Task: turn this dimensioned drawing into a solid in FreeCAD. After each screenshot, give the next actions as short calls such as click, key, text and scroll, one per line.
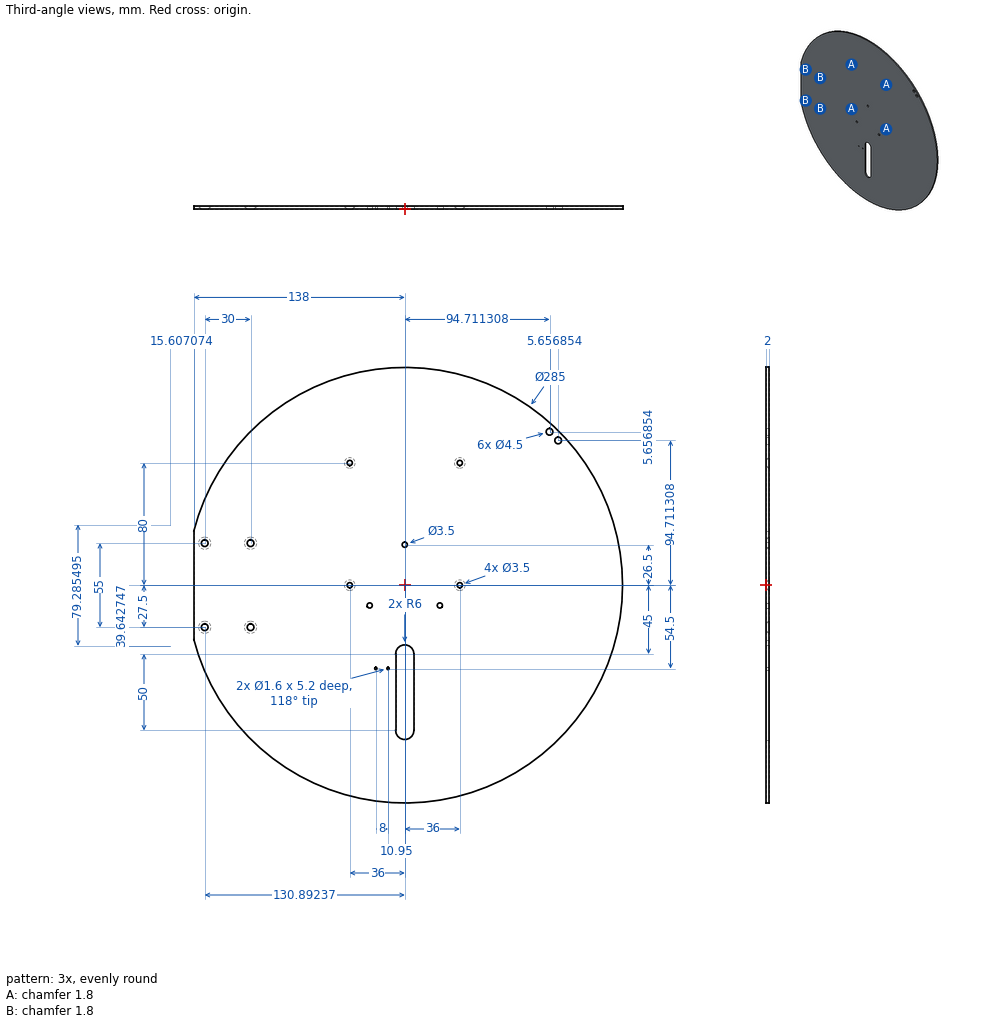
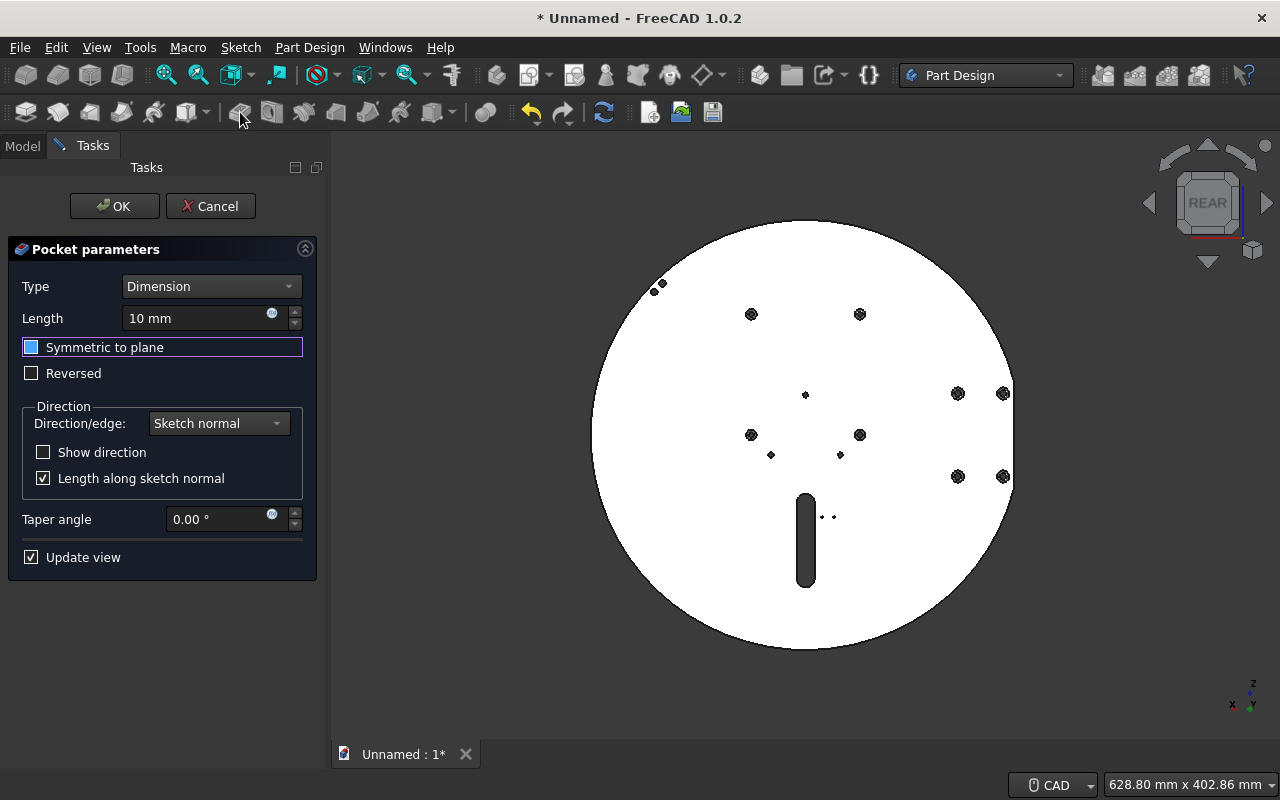
click(115, 206)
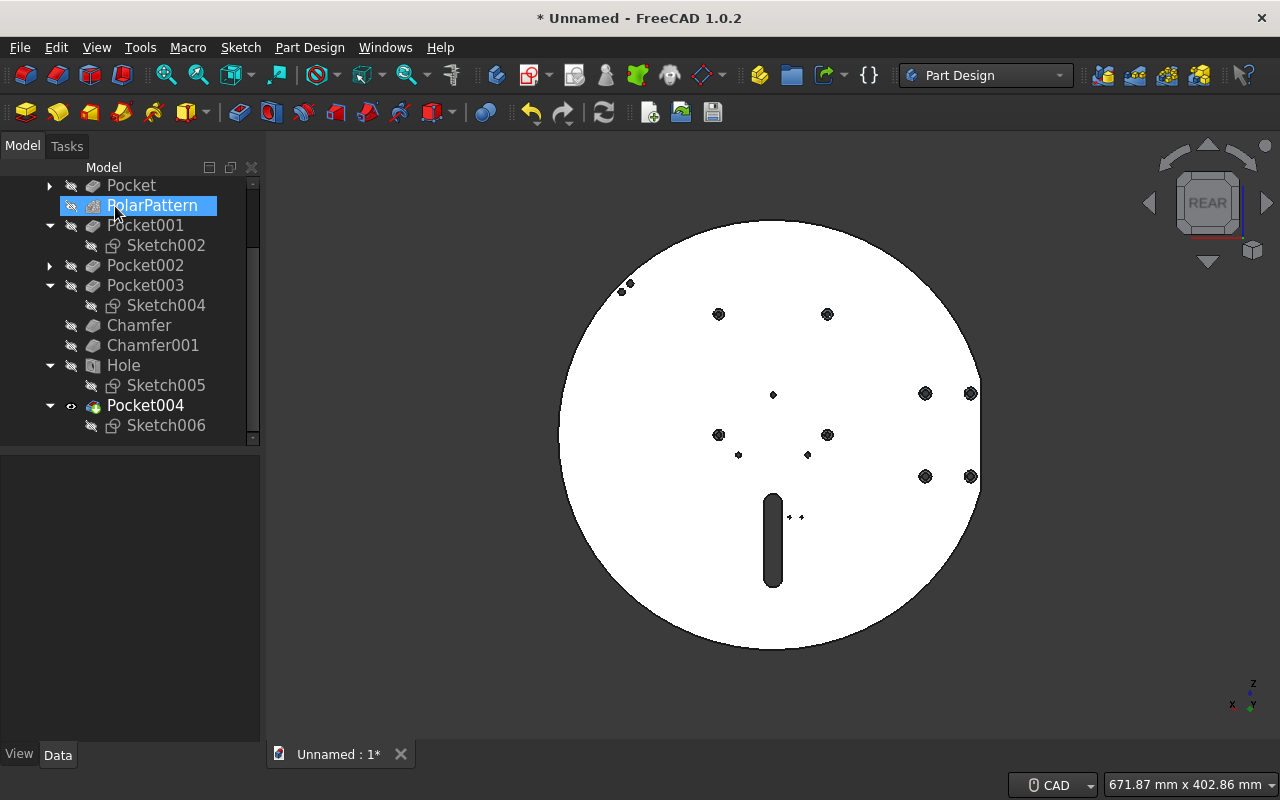
key(0)